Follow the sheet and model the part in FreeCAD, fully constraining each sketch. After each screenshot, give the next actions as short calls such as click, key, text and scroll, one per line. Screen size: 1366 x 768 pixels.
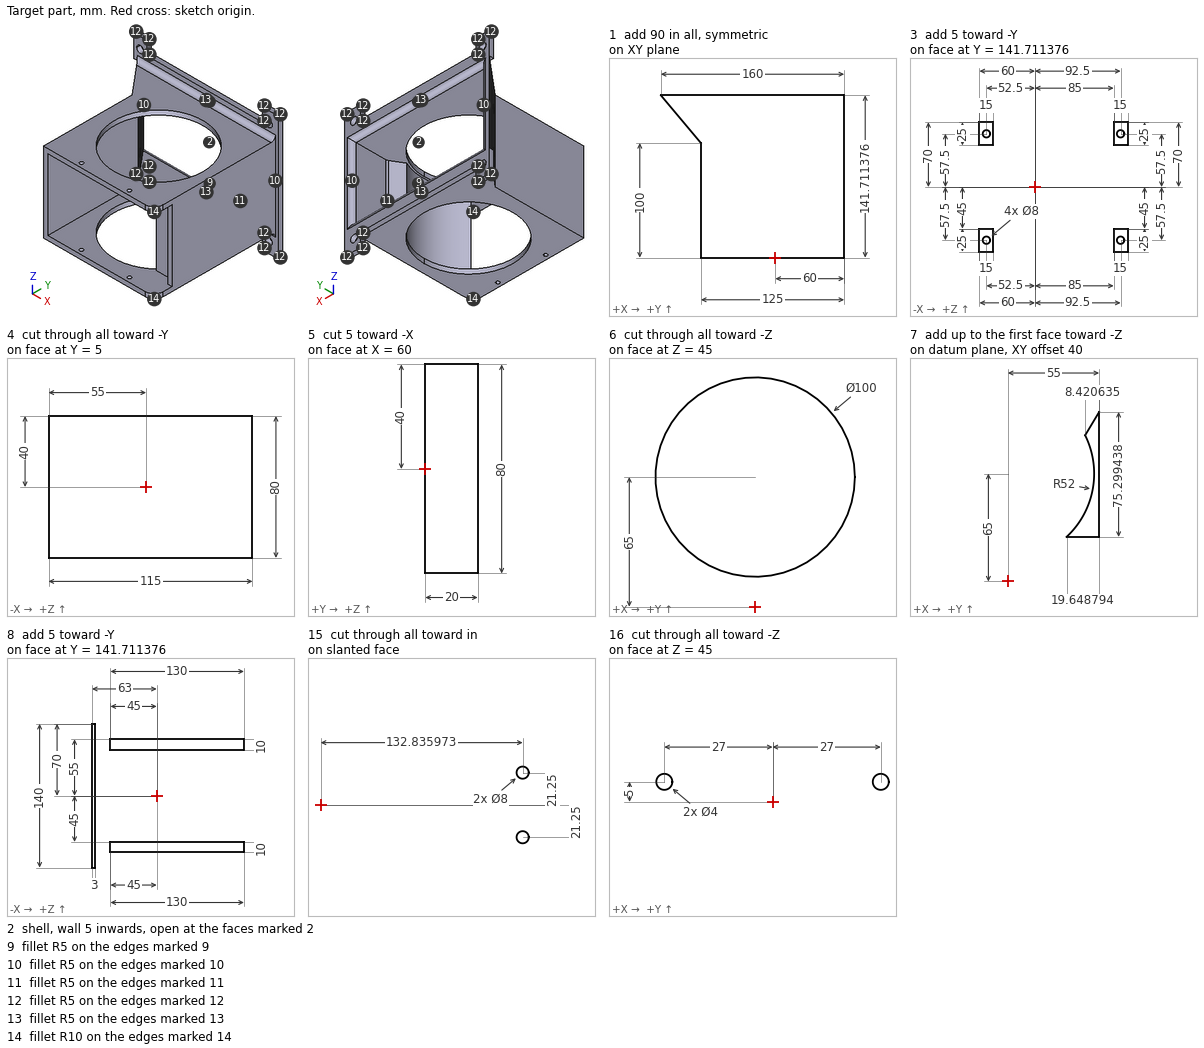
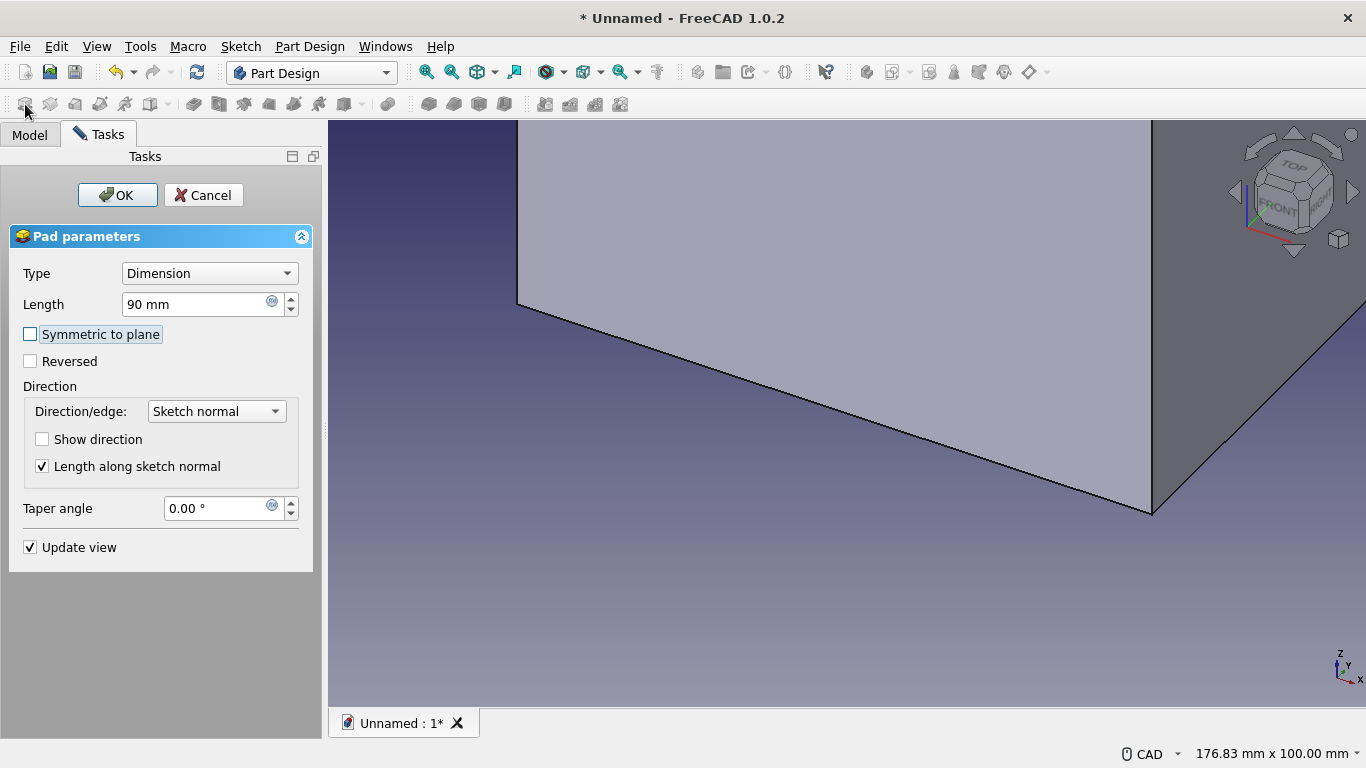
click(31, 334)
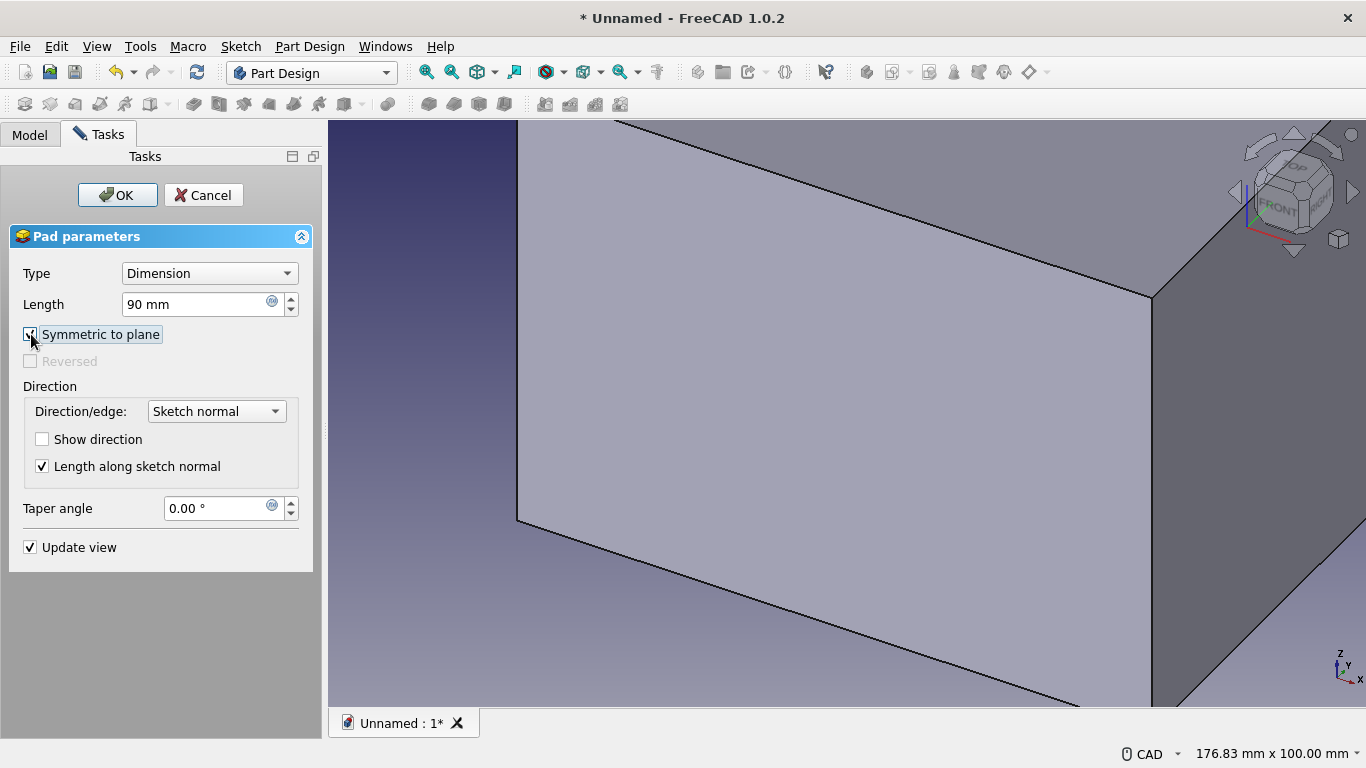
click(118, 195)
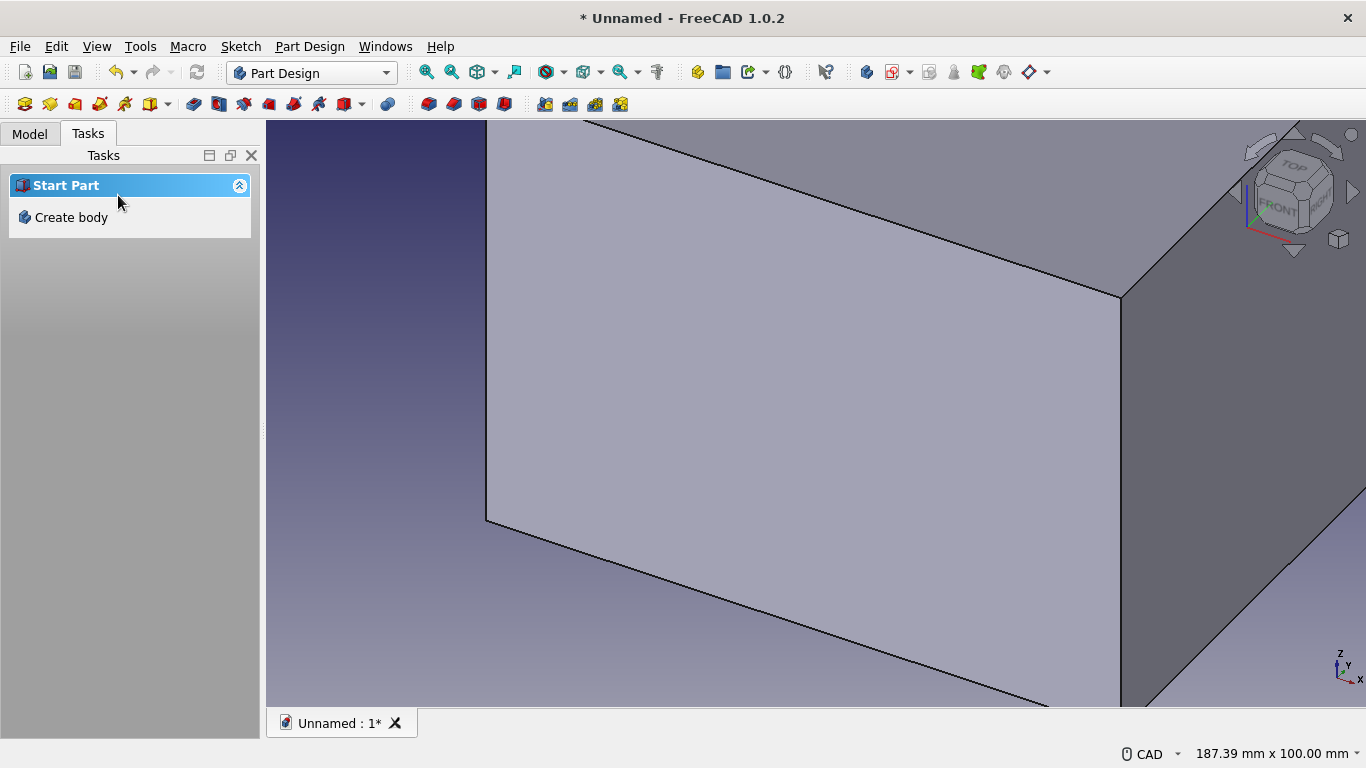
key(v)
key(f)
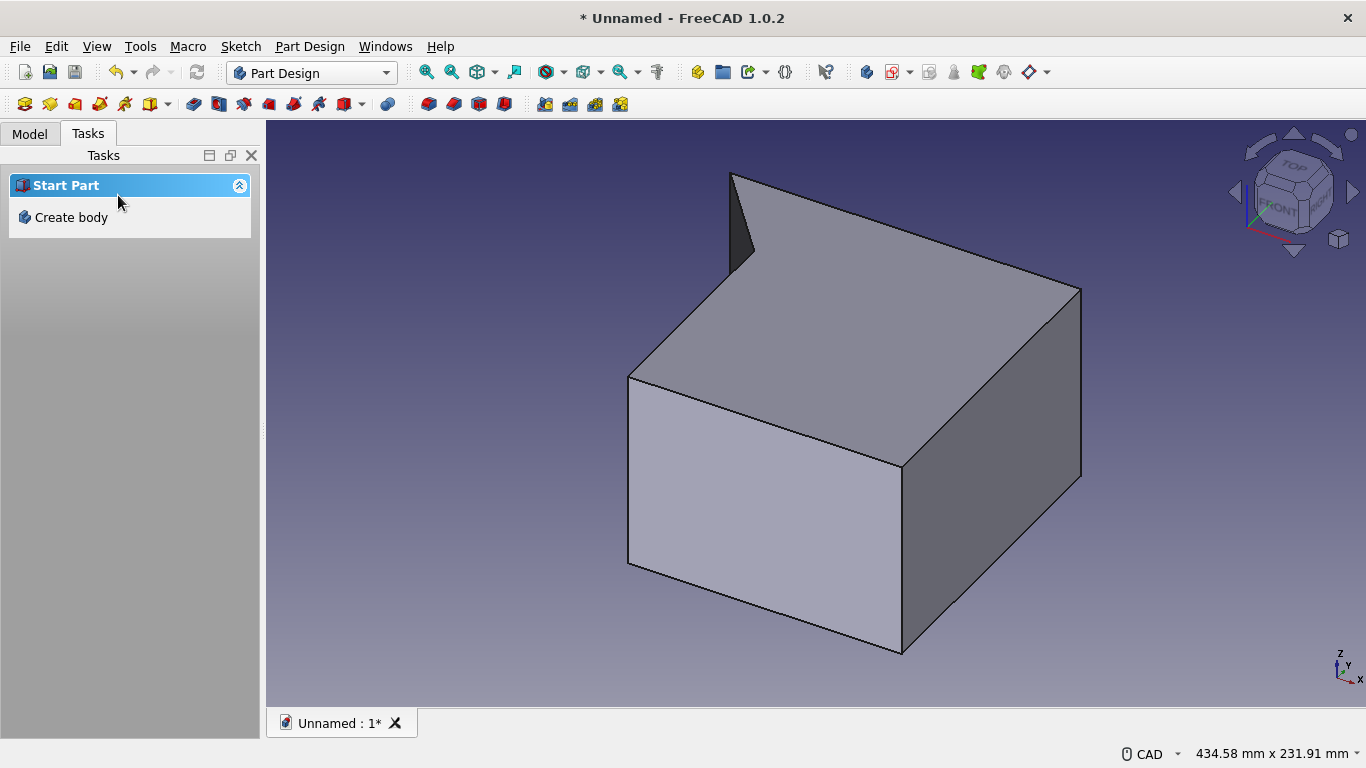
key(0)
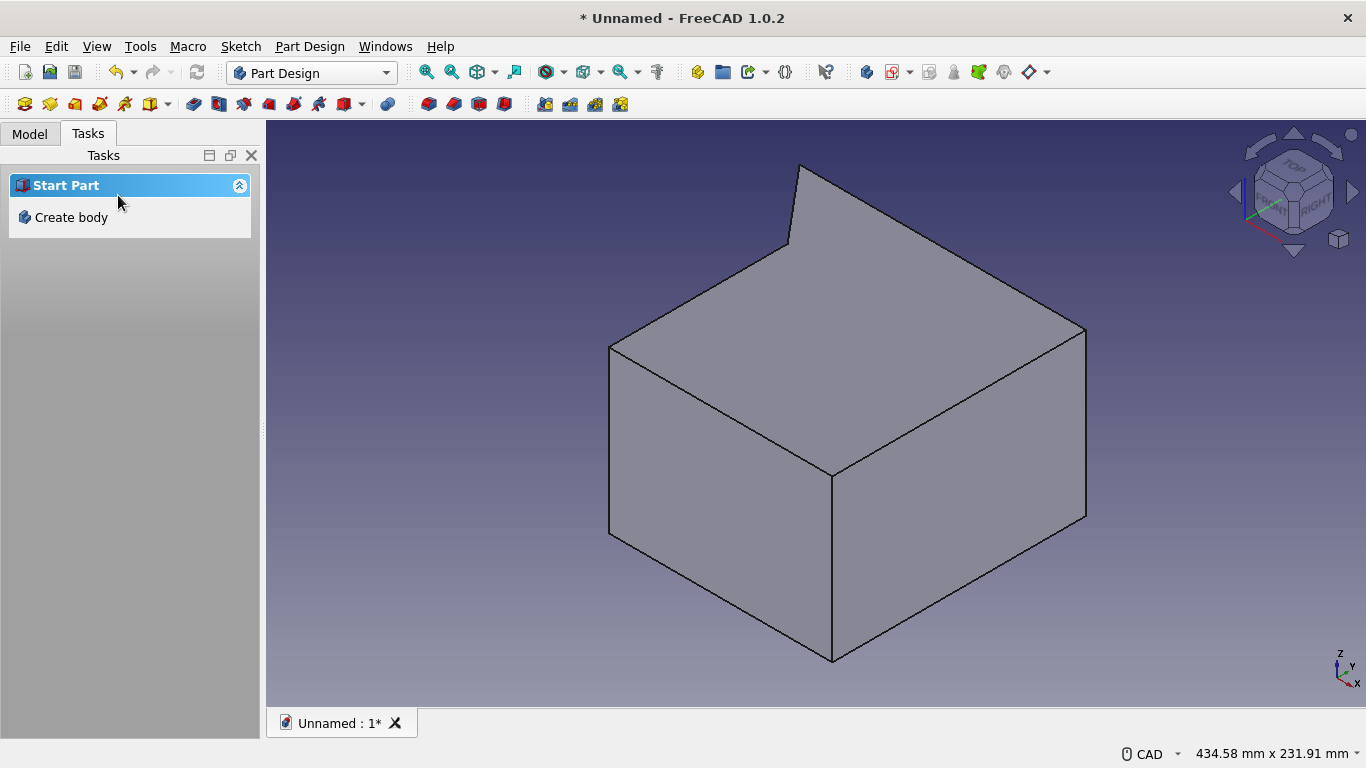
key(2)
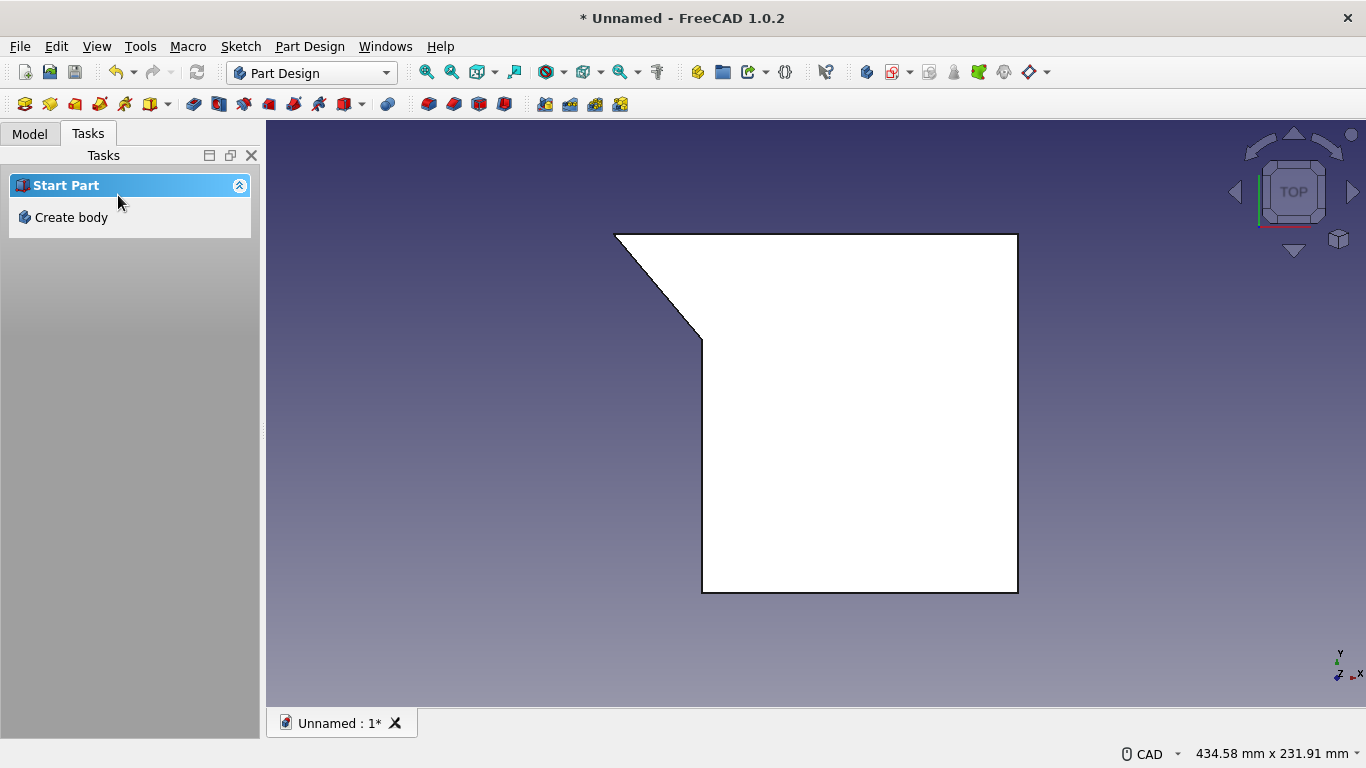
key(1)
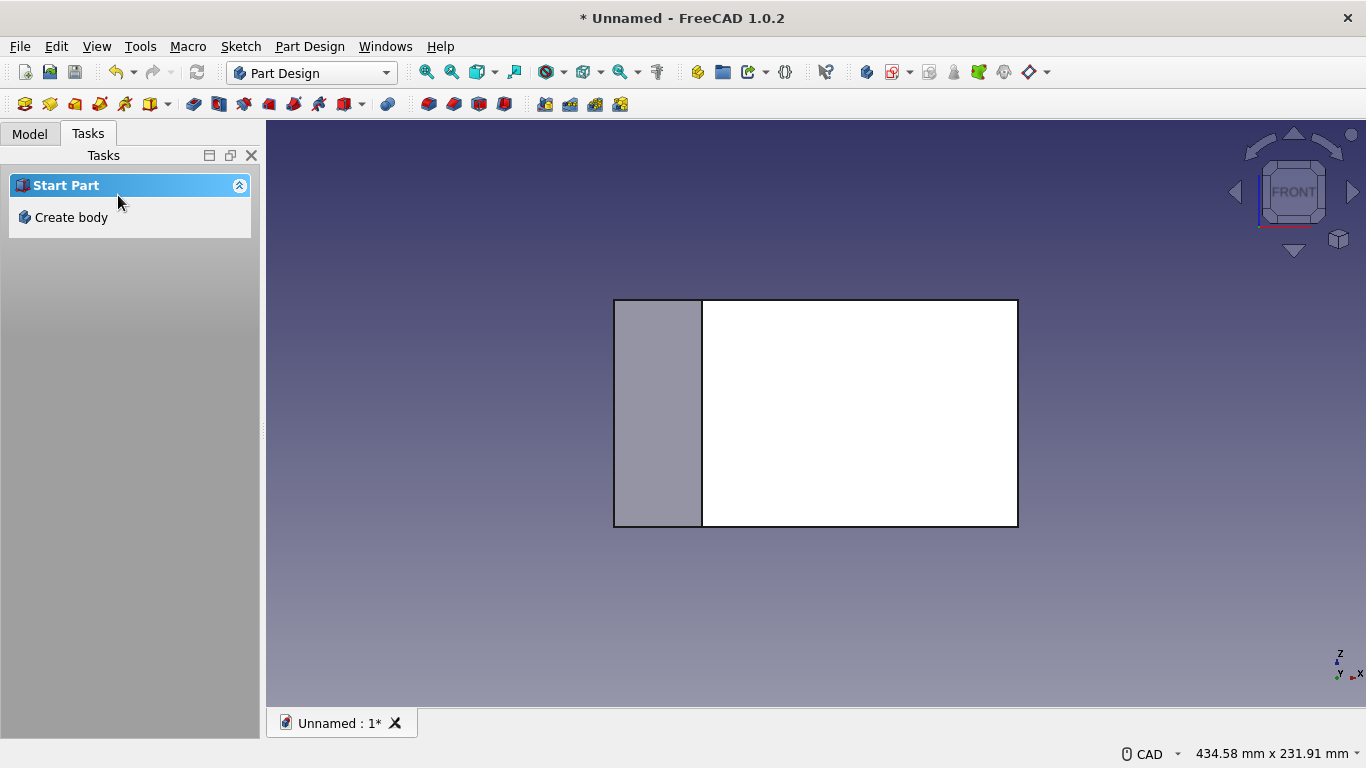
key(v)
key(f)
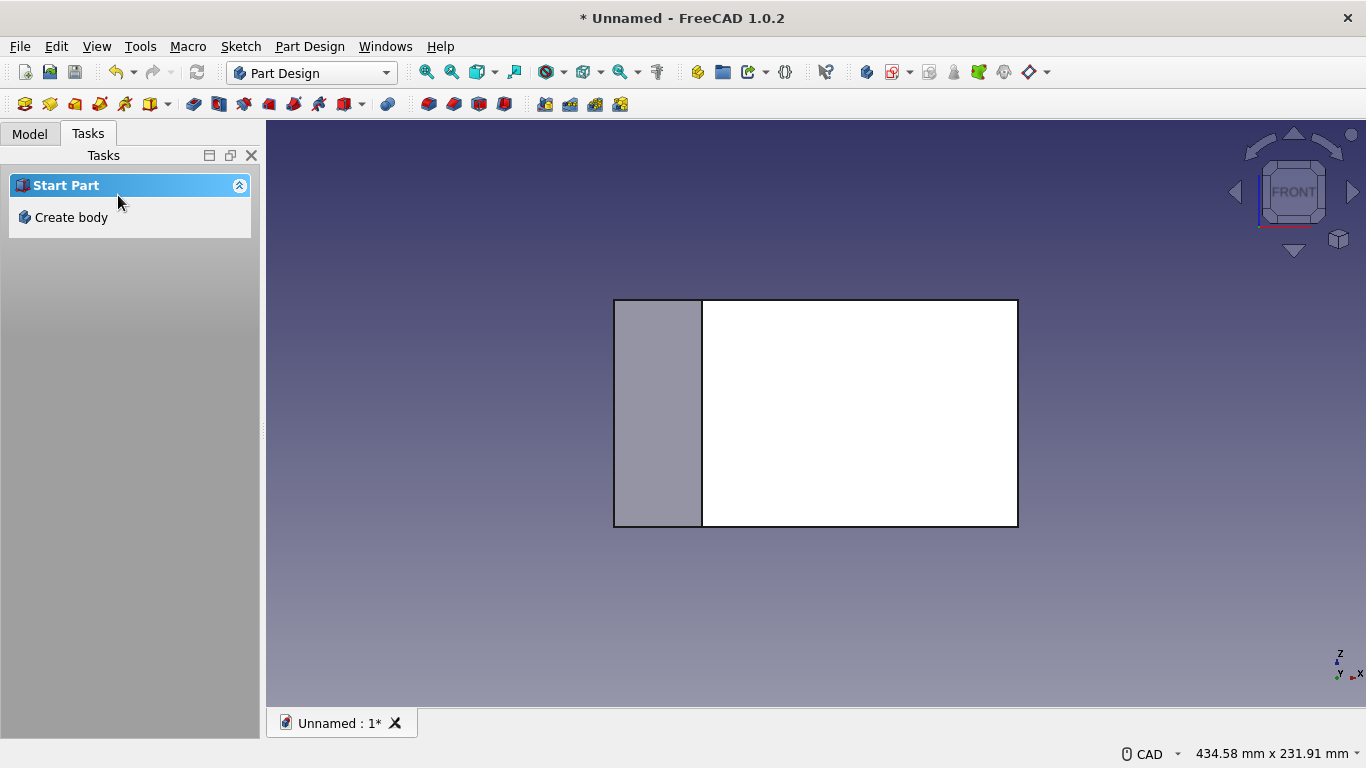
key(3)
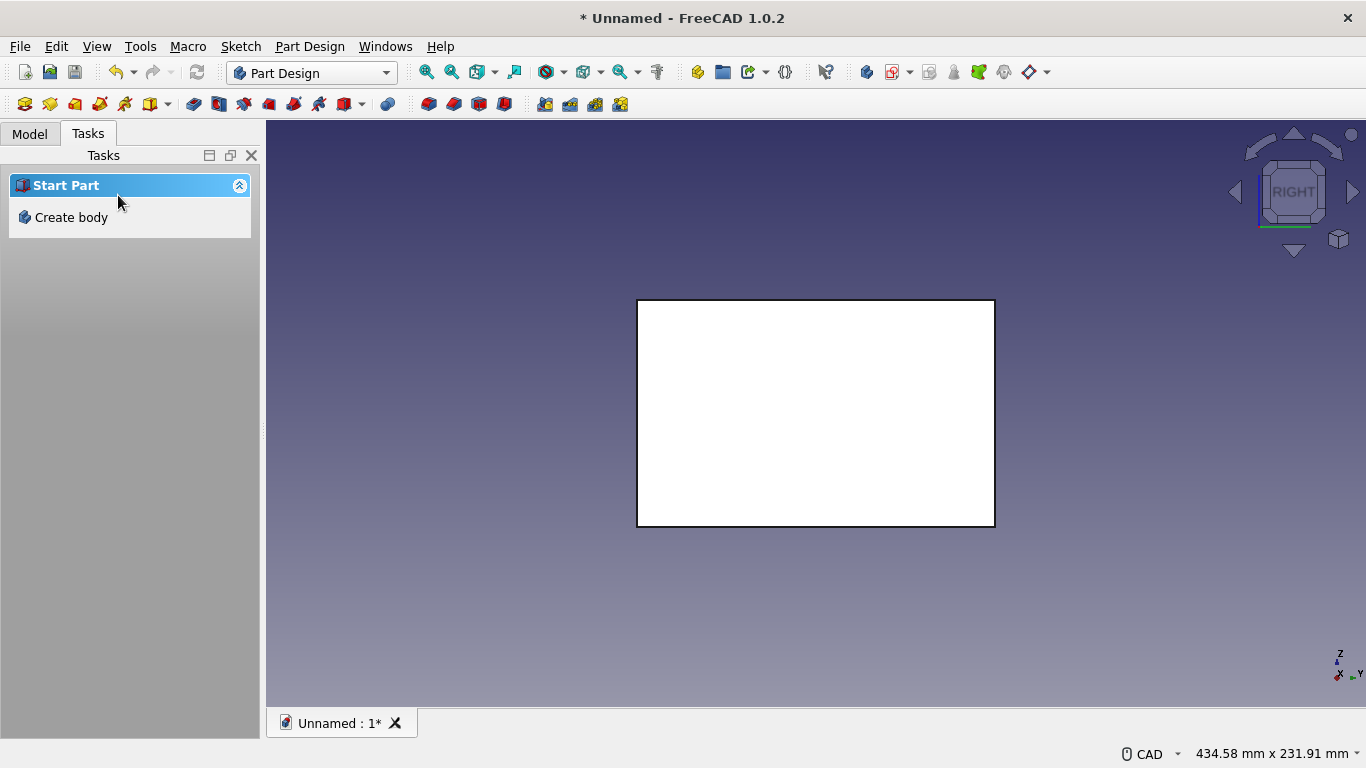
key(v)
key(f)